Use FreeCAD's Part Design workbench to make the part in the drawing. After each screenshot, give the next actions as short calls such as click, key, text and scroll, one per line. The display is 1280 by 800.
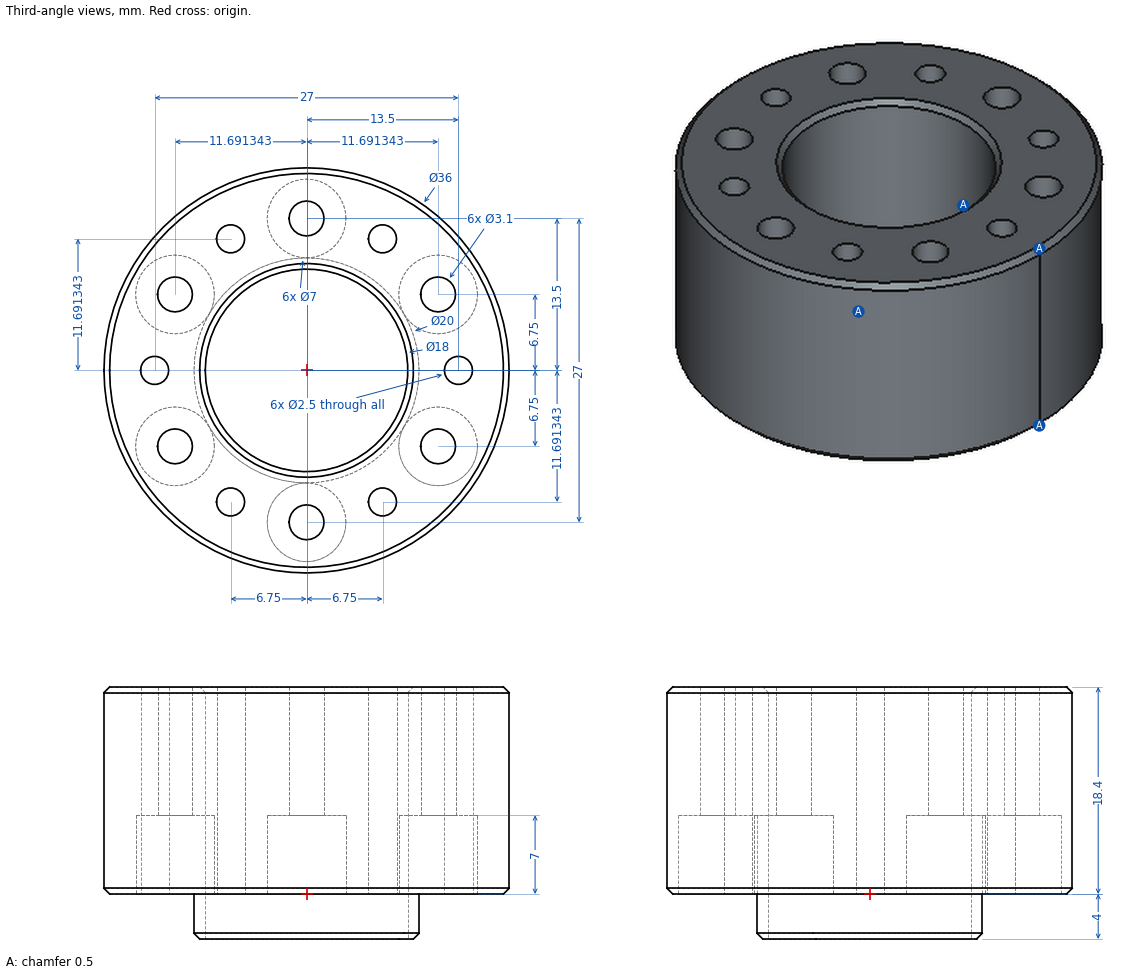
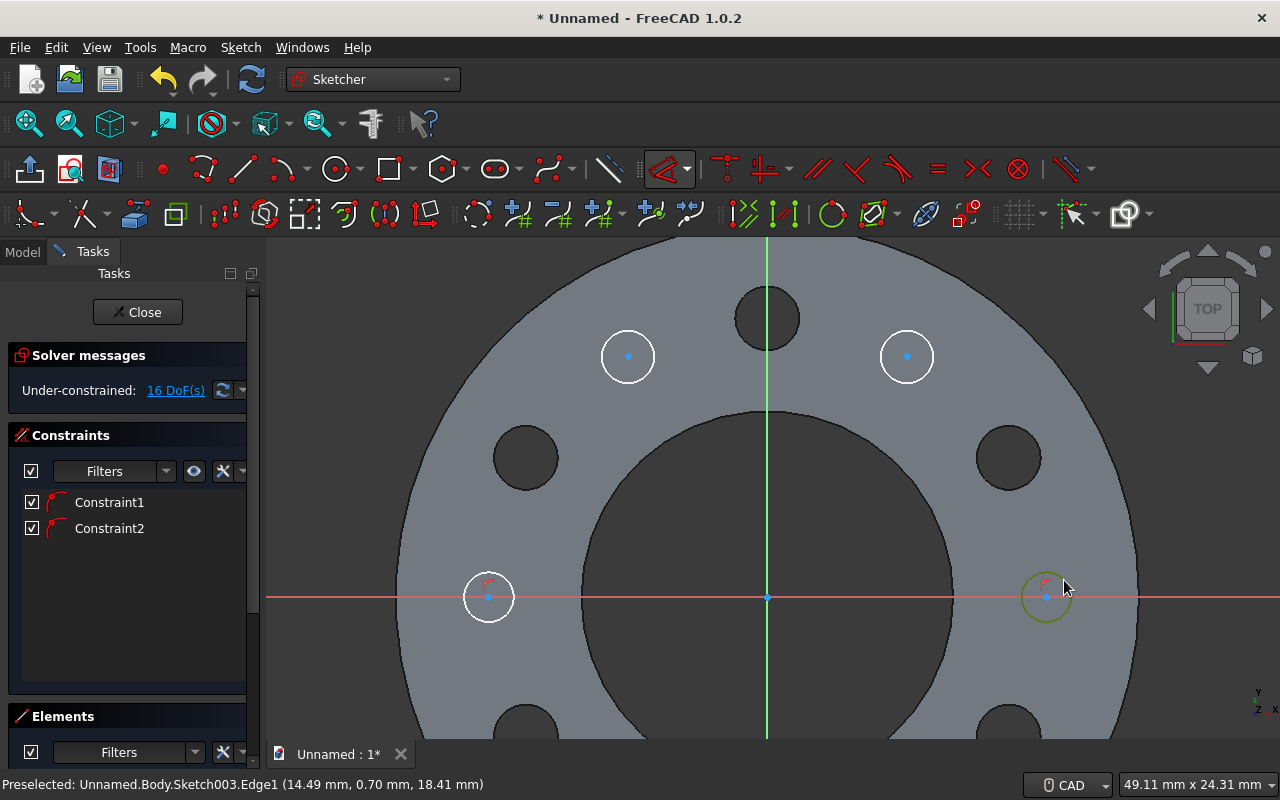
scroll(628, 355, down, 3)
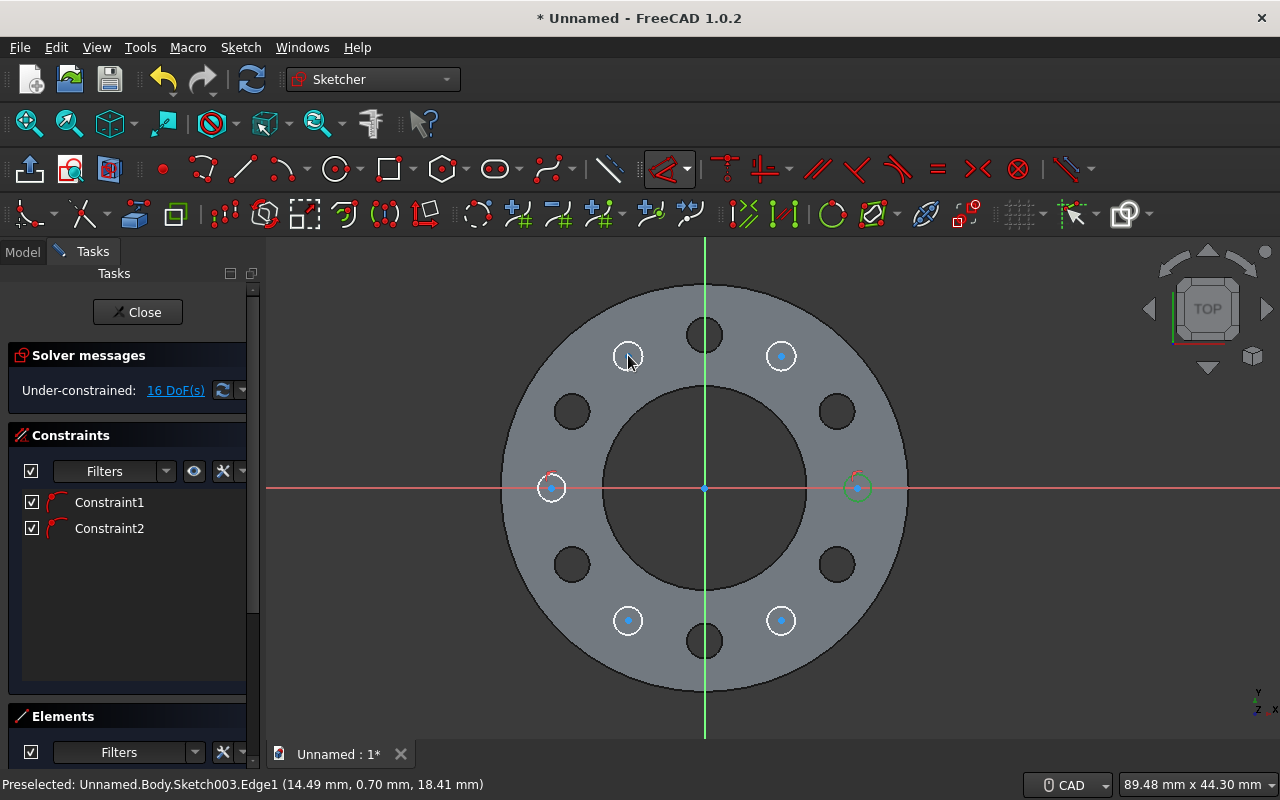
click(791, 611)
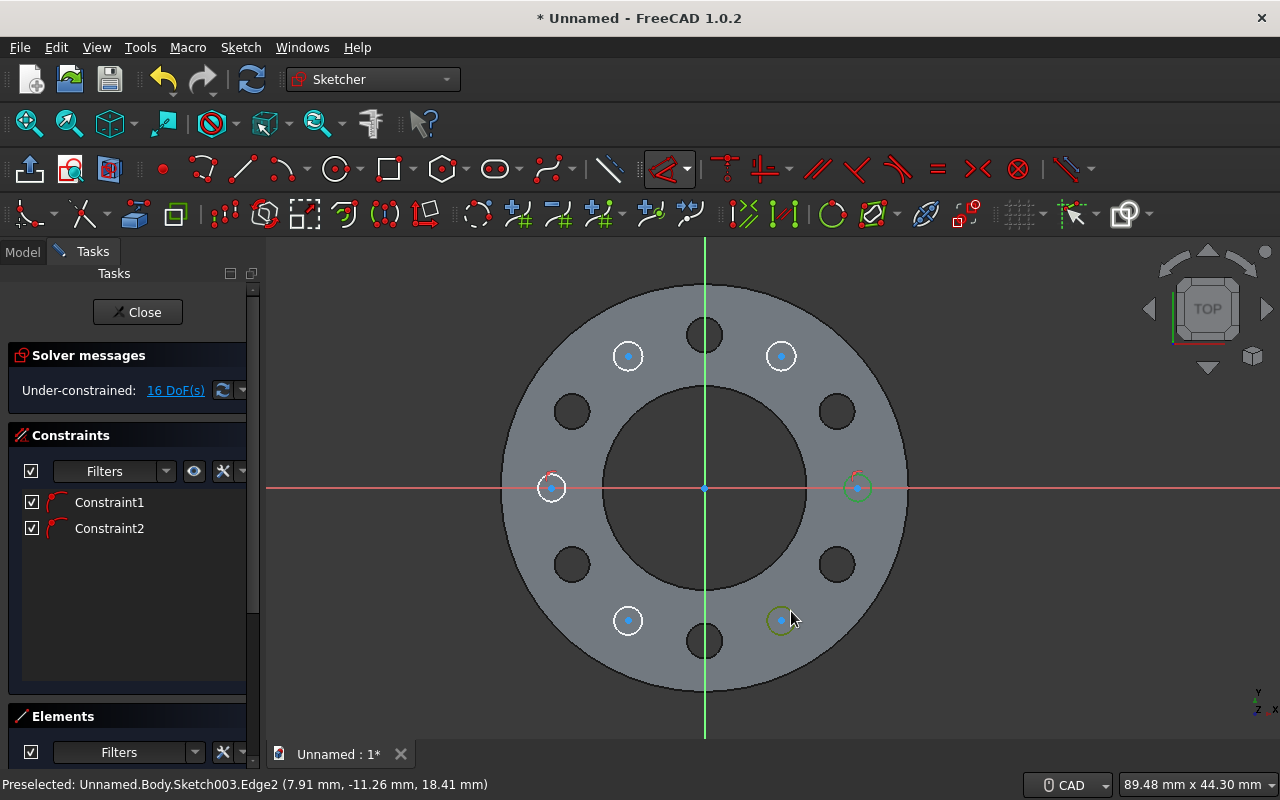
click(638, 611)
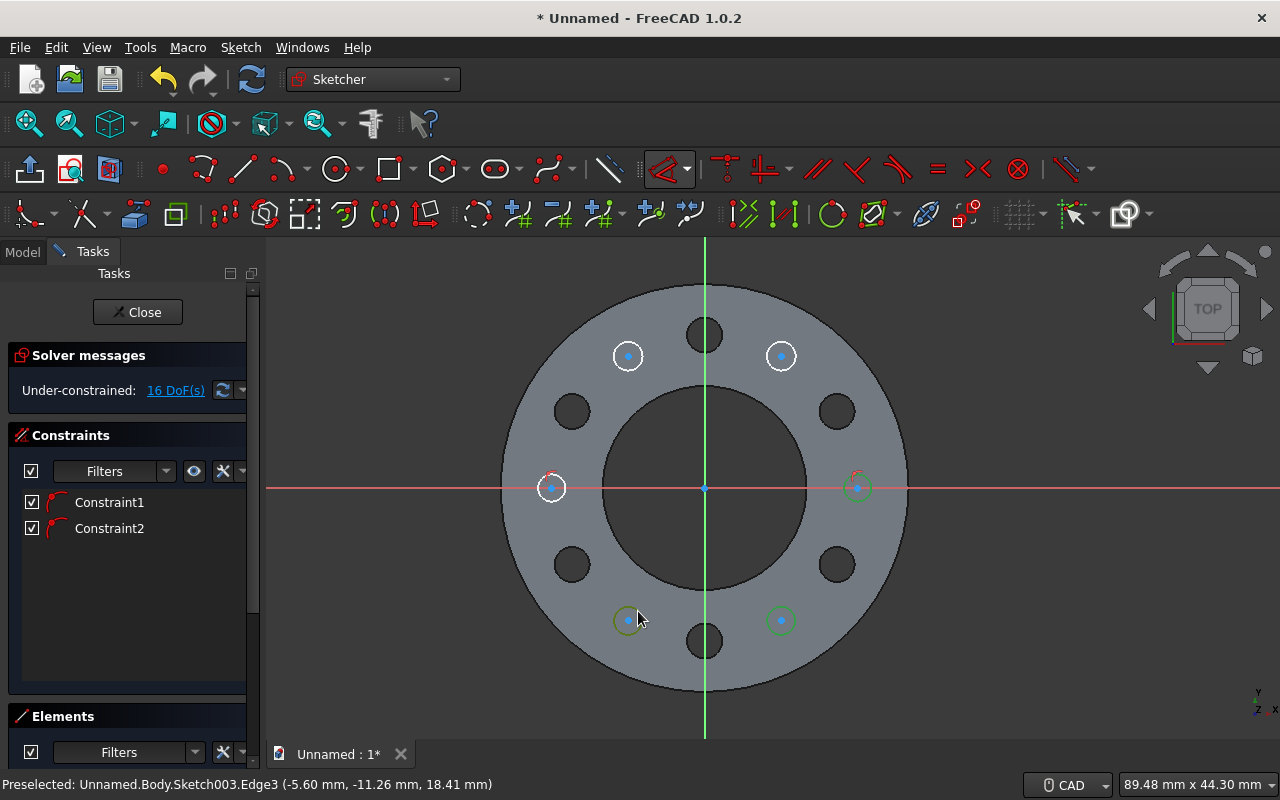
scroll(561, 478, up, 2)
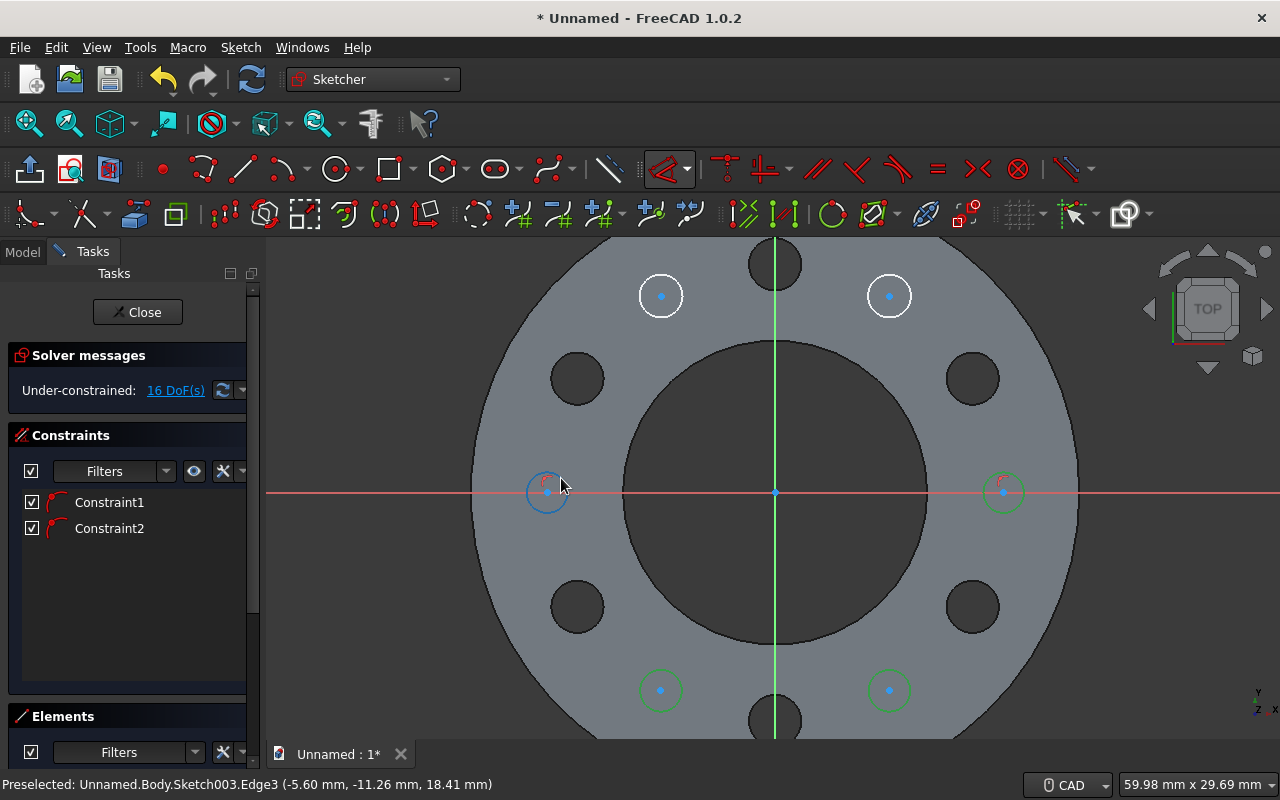
click(561, 478)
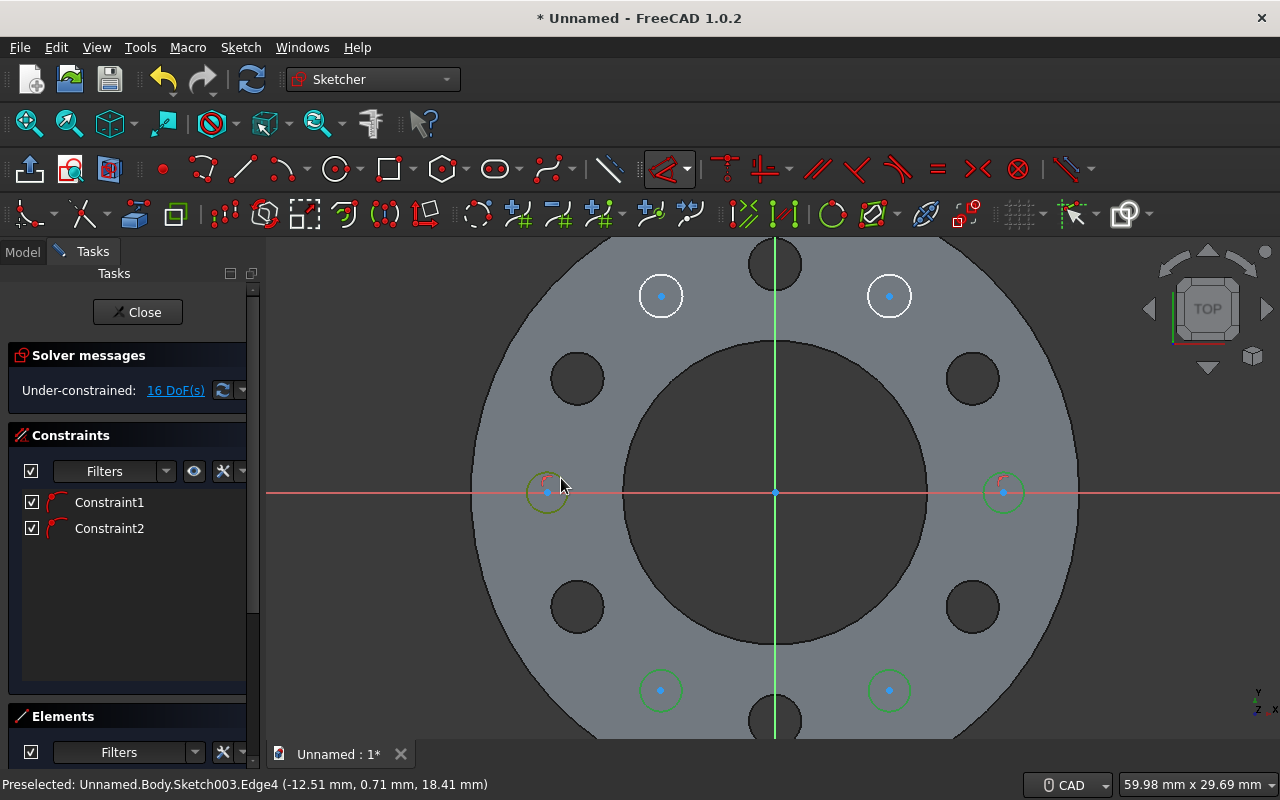
click(676, 281)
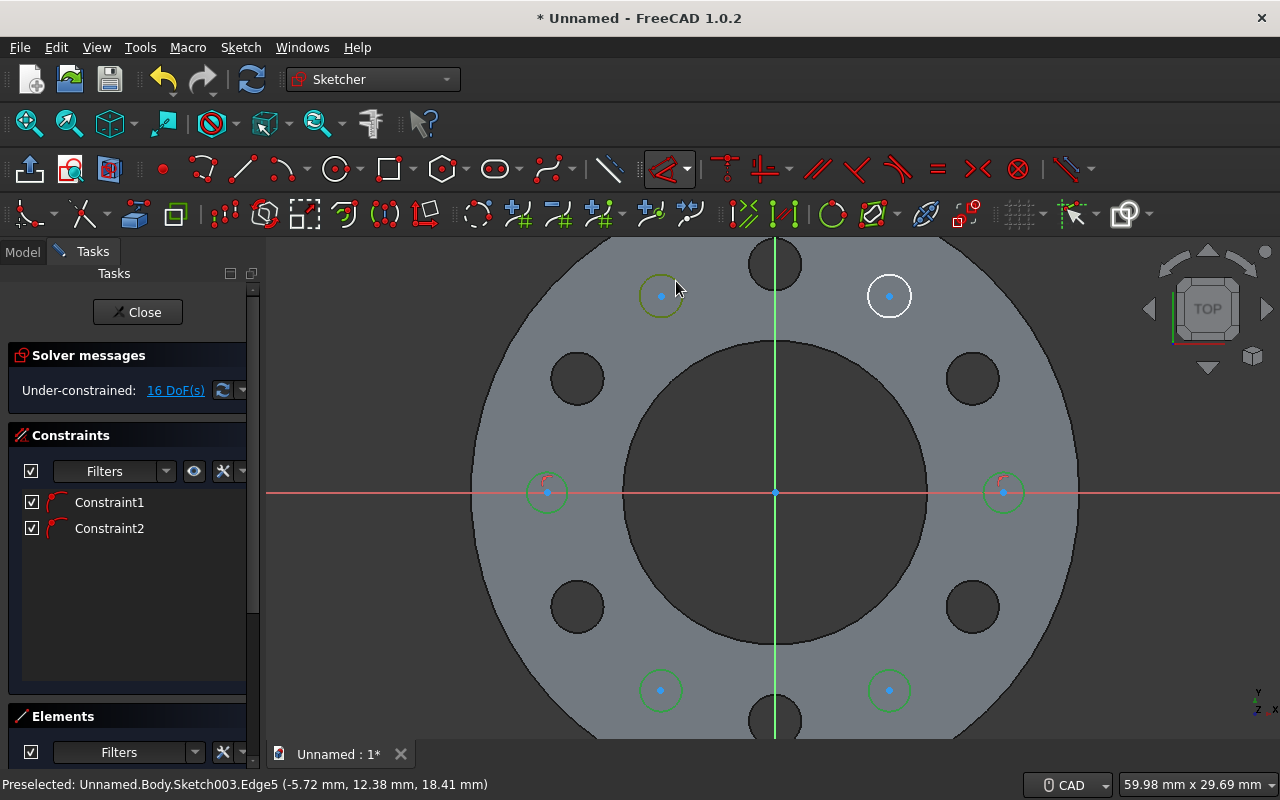
click(905, 281)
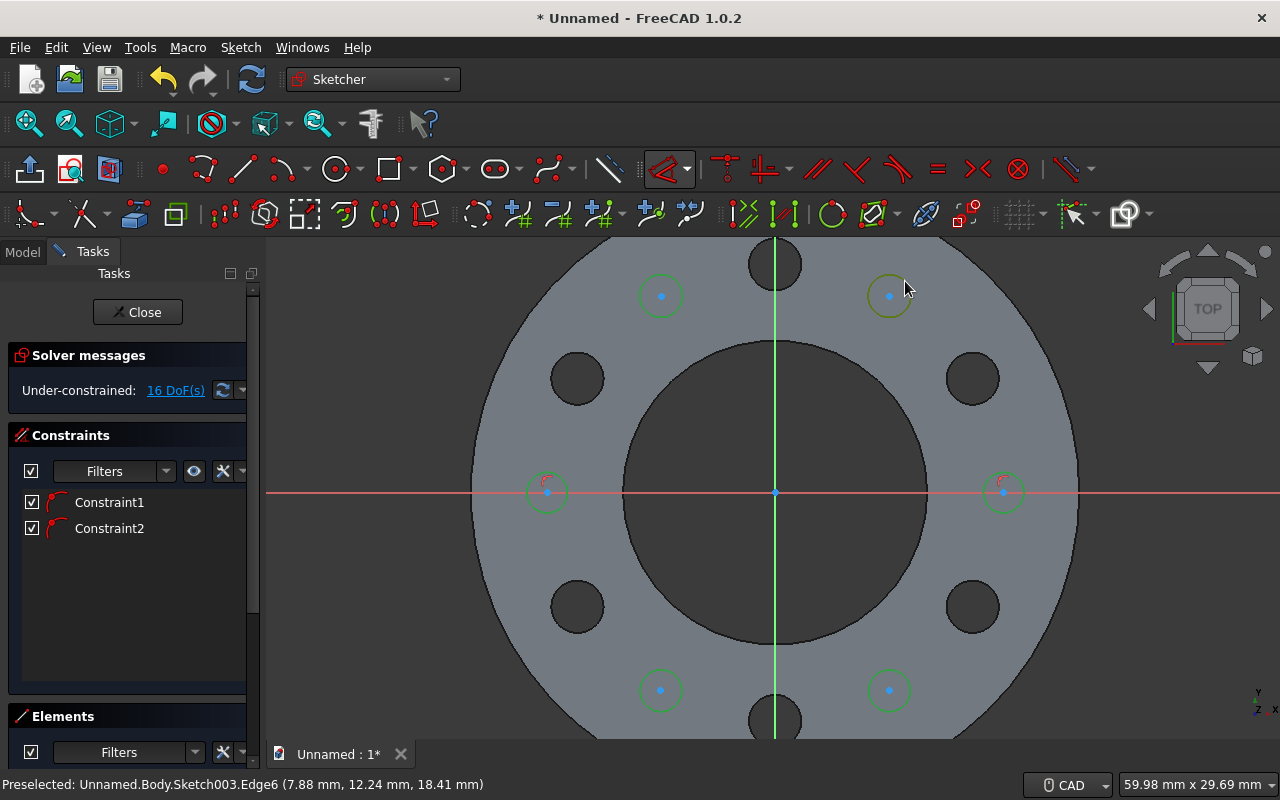
click(938, 170)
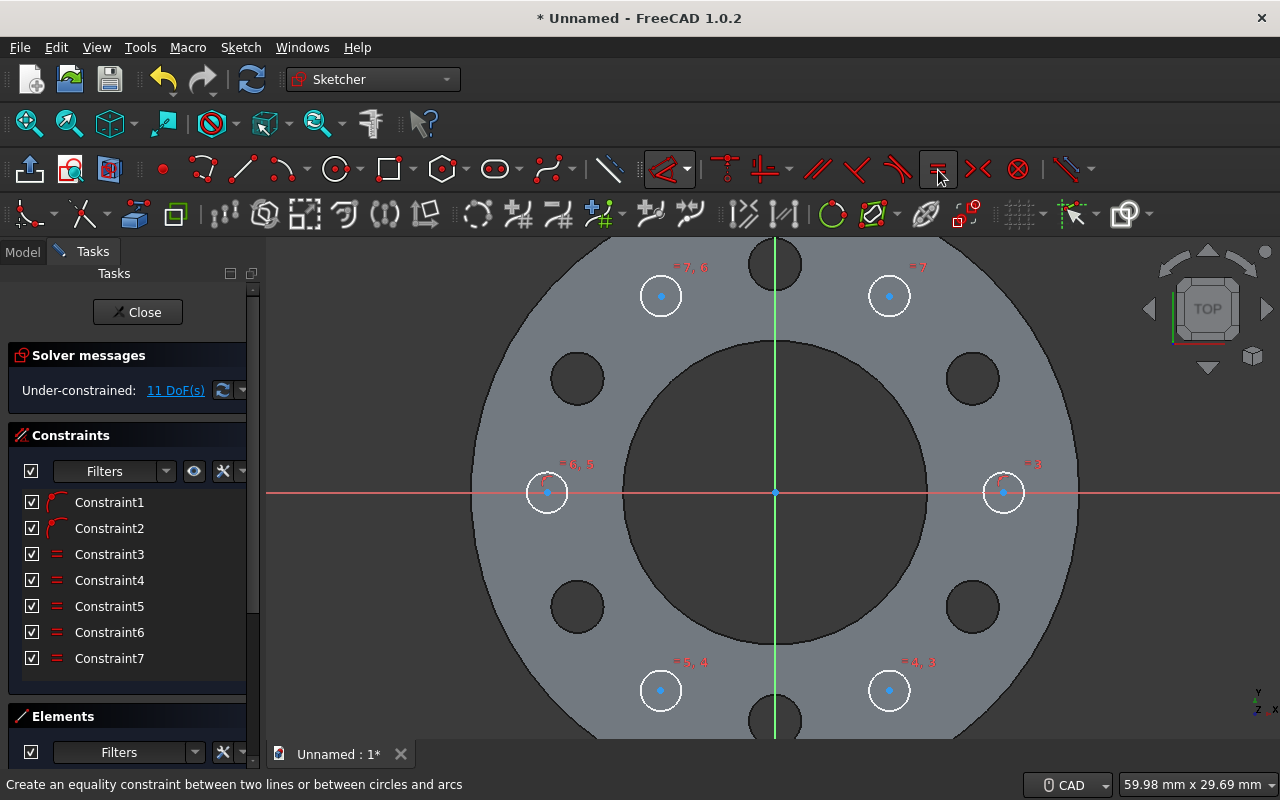
click(1018, 478)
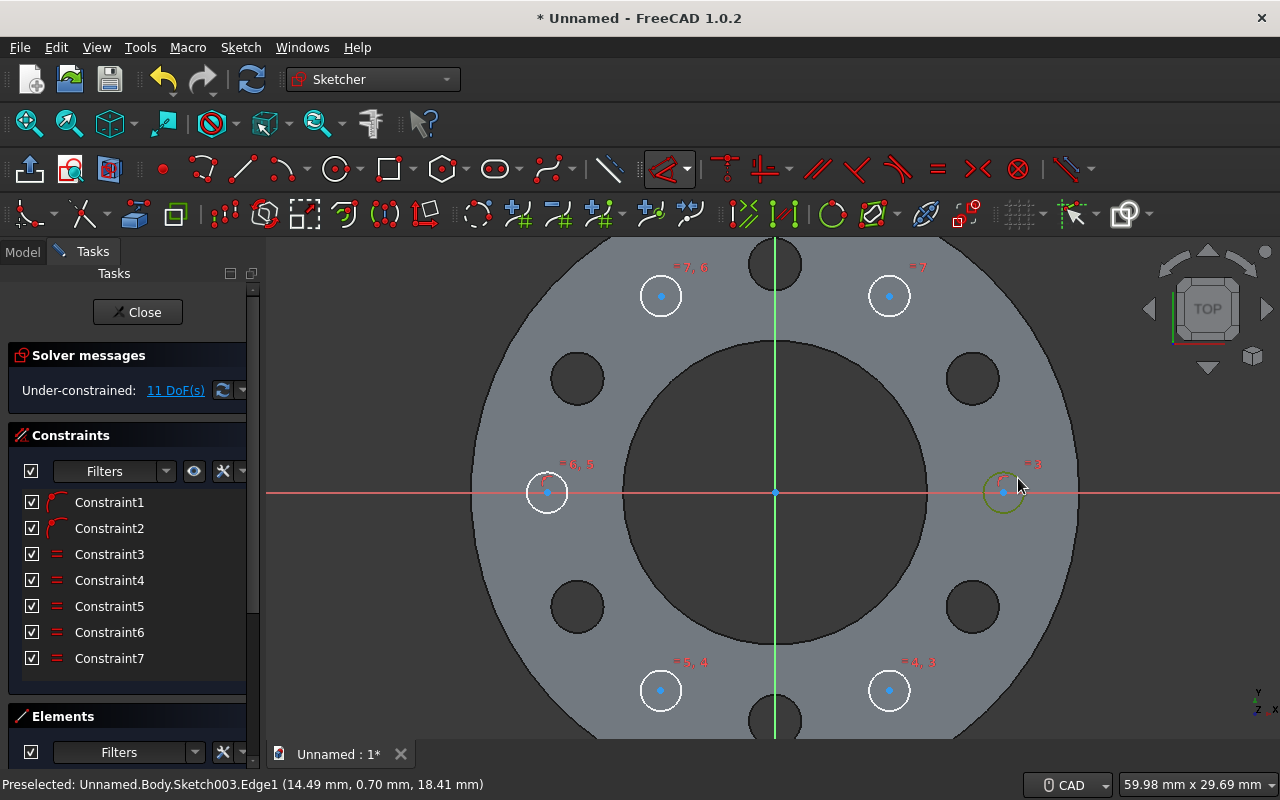
click(690, 170)